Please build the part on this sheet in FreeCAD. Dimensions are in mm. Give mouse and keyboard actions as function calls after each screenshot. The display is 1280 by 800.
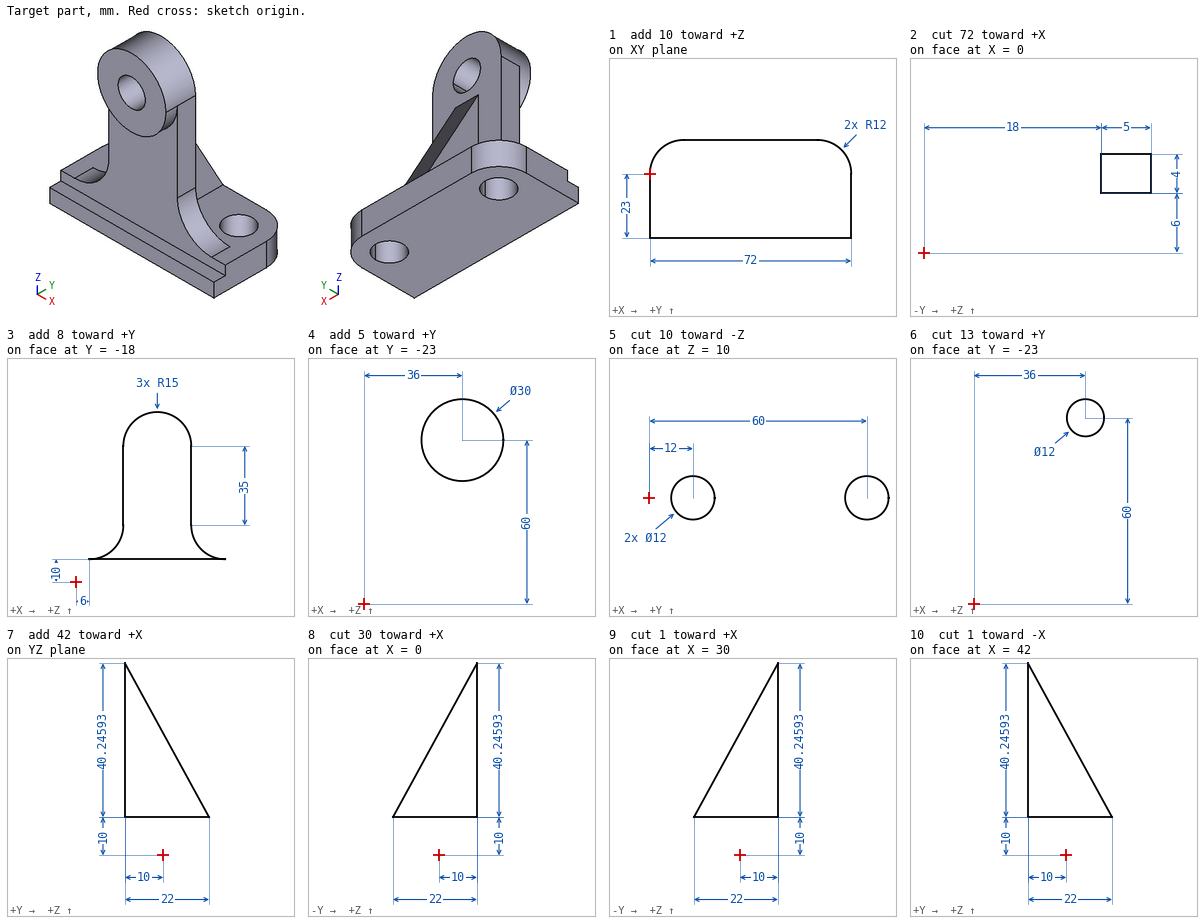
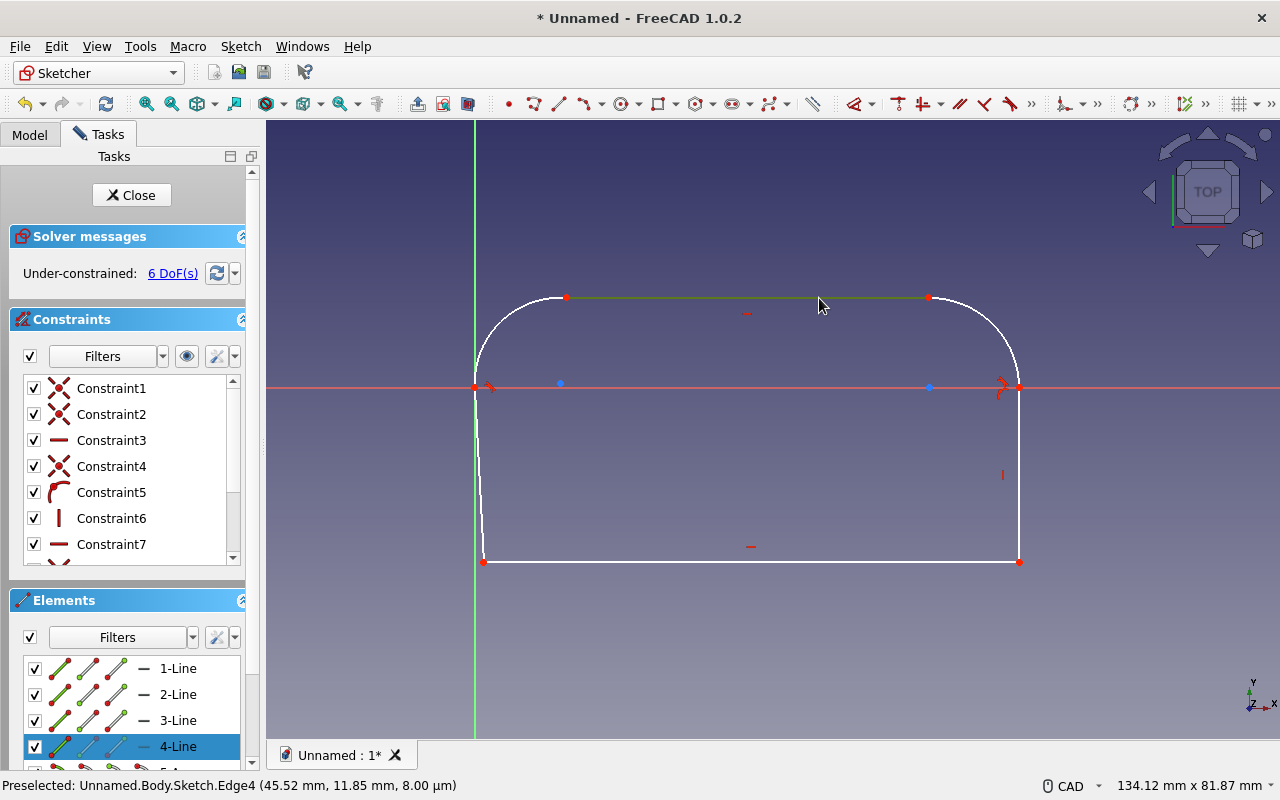
click(1009, 347)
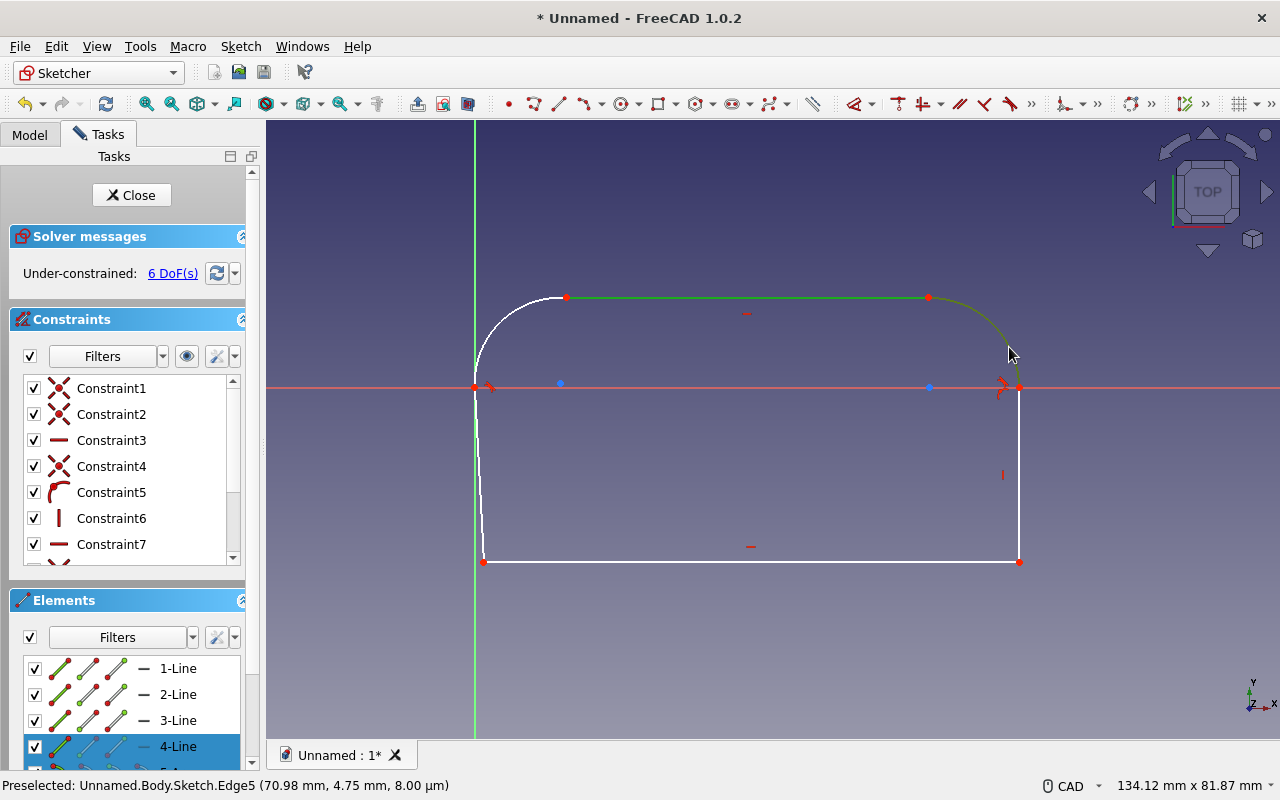
click(1010, 104)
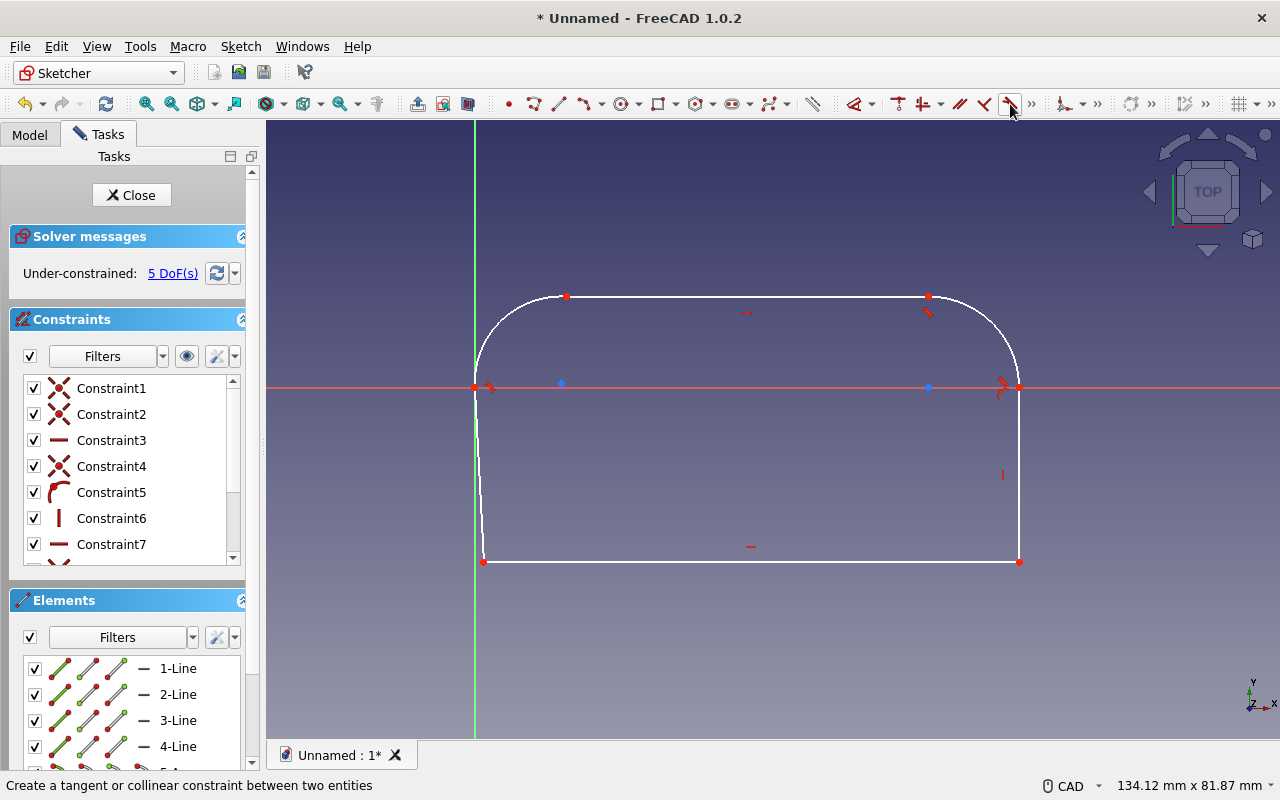
click(819, 297)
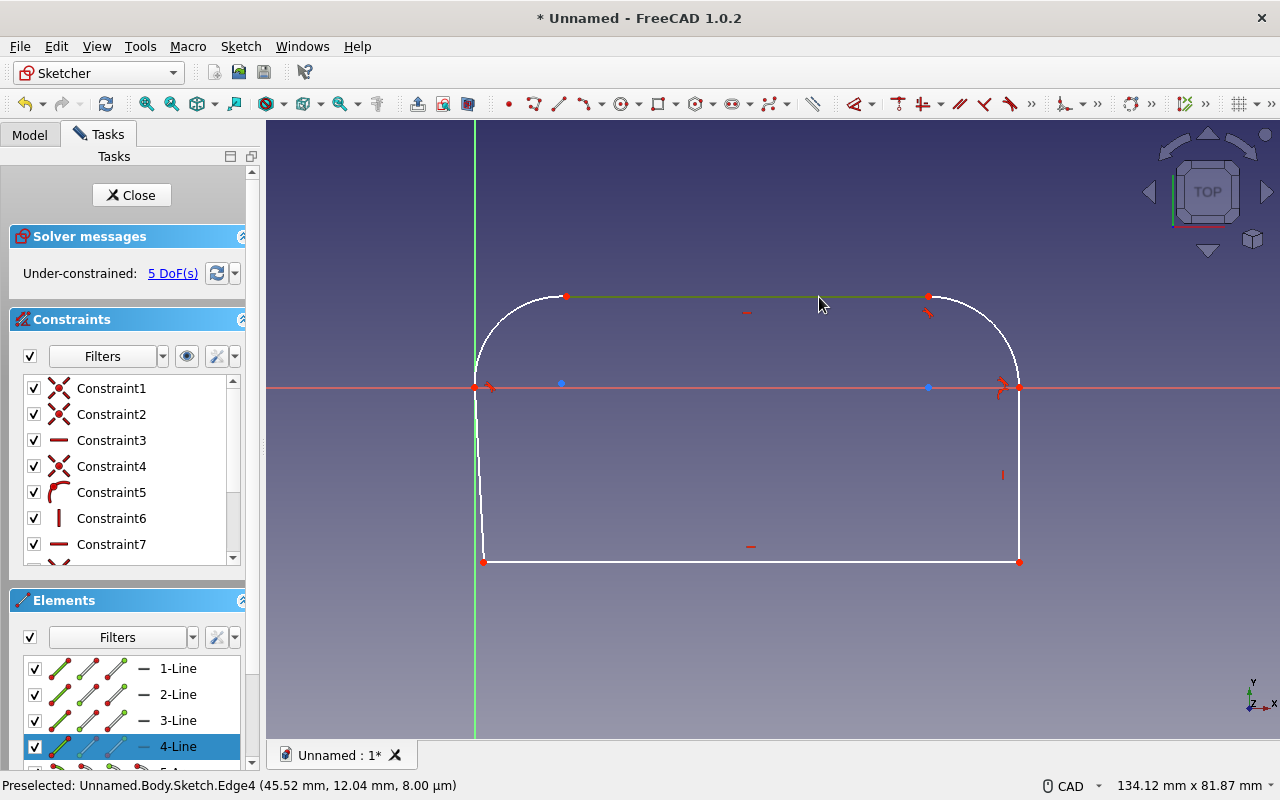
click(524, 305)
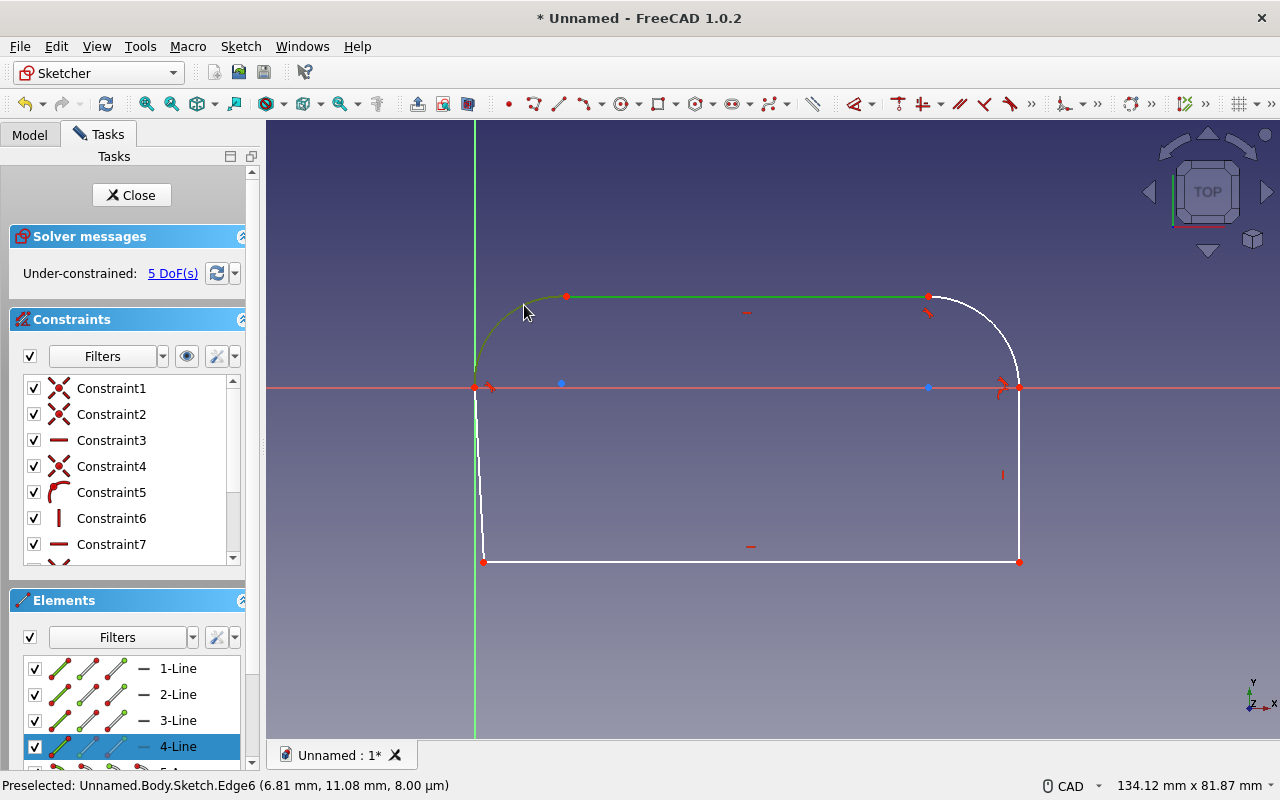
click(1010, 104)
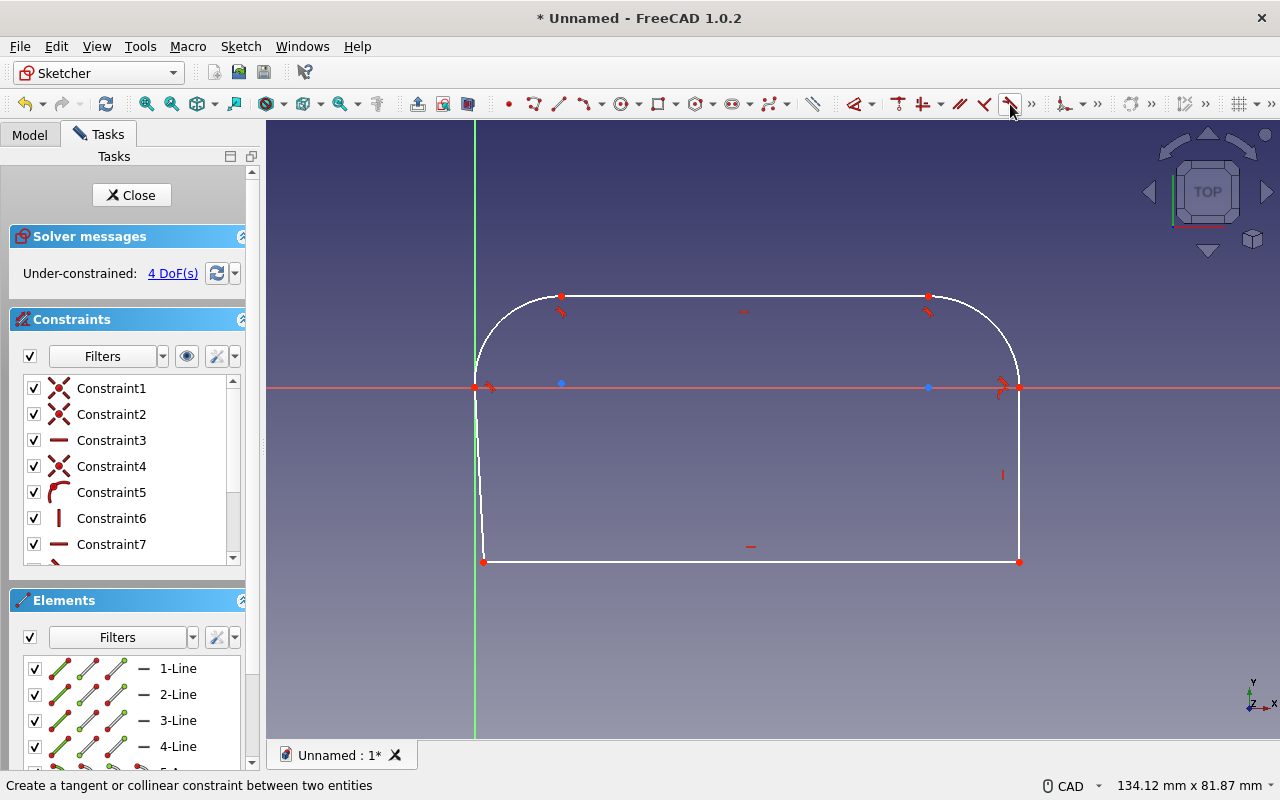
click(478, 440)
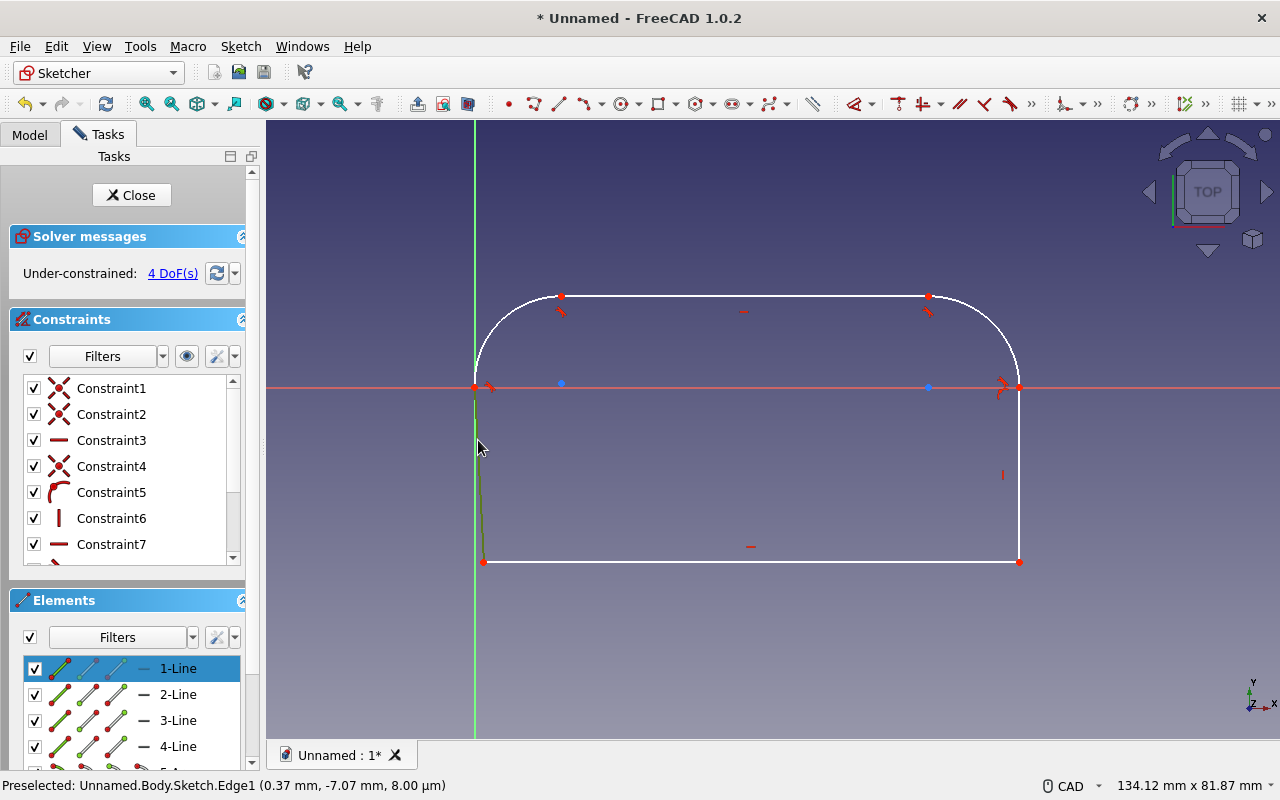
click(940, 104)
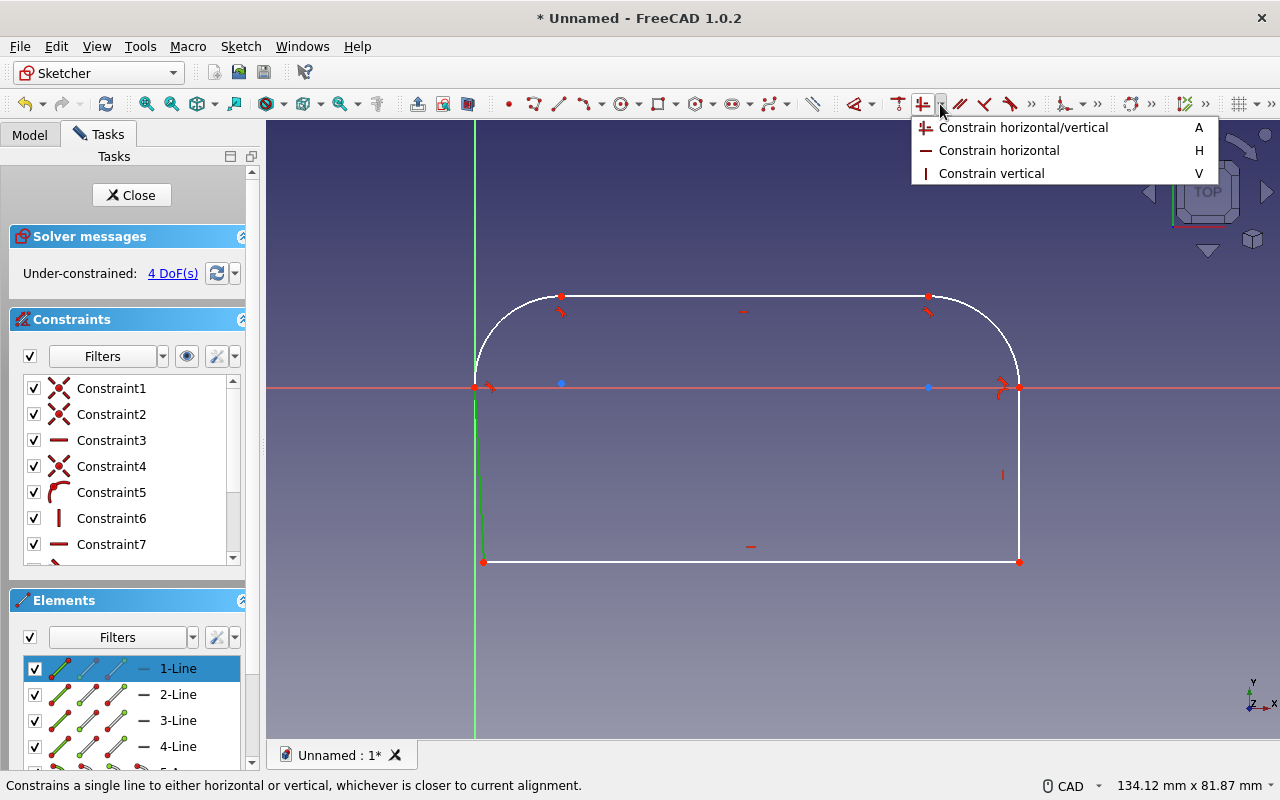
click(1065, 174)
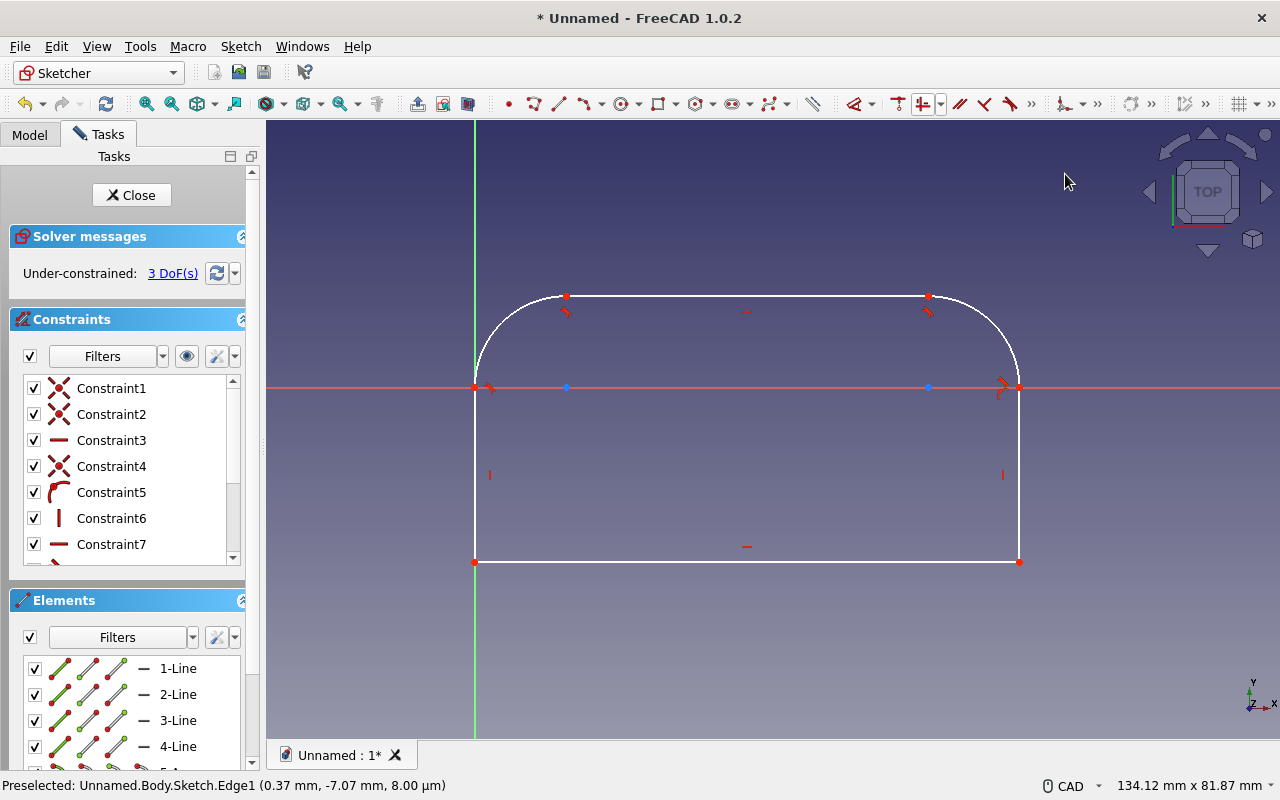
click(1009, 346)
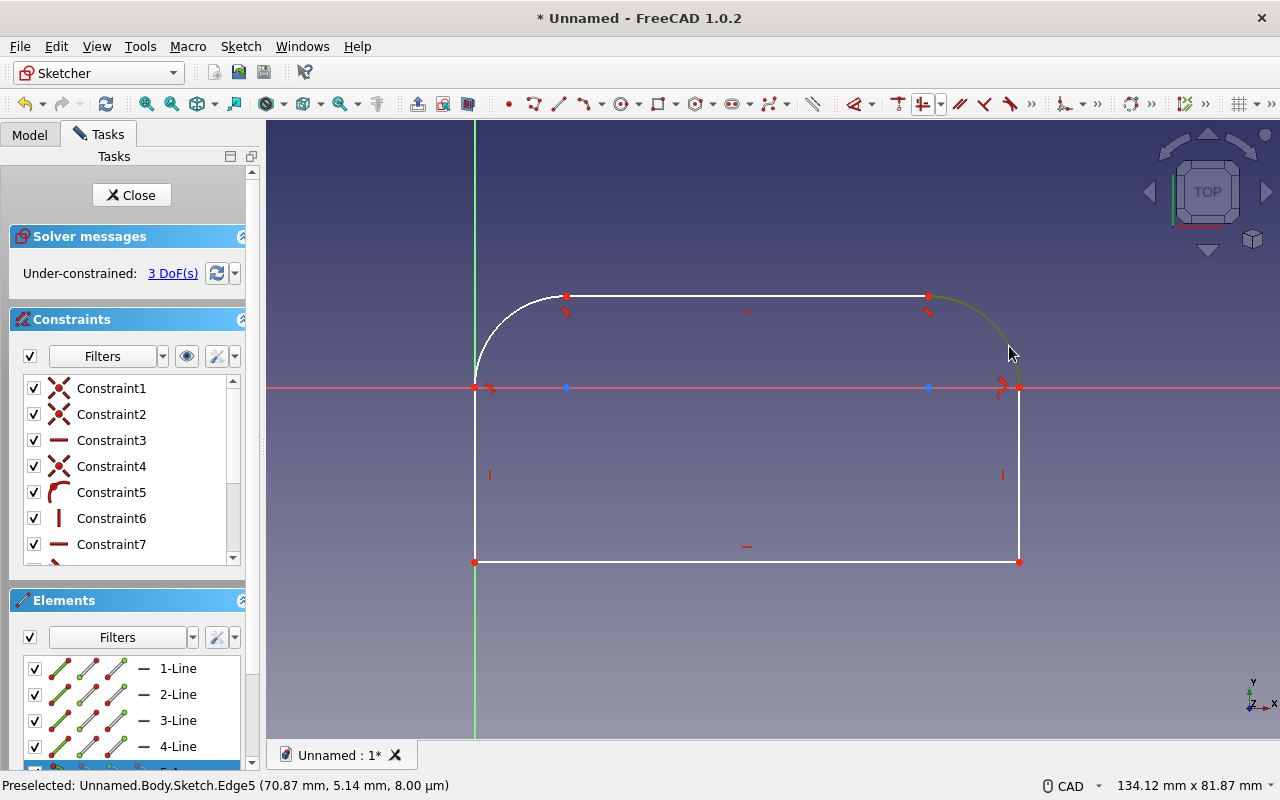
key(k)
key(r)